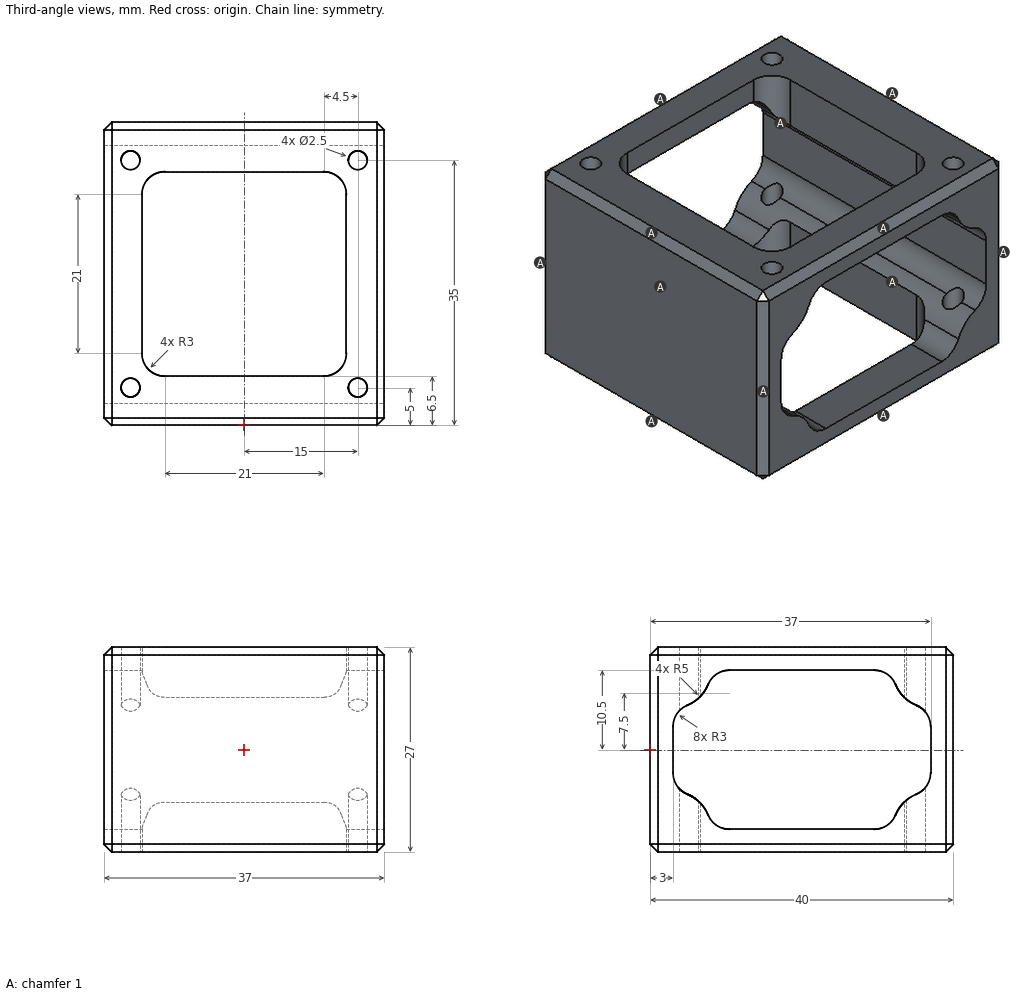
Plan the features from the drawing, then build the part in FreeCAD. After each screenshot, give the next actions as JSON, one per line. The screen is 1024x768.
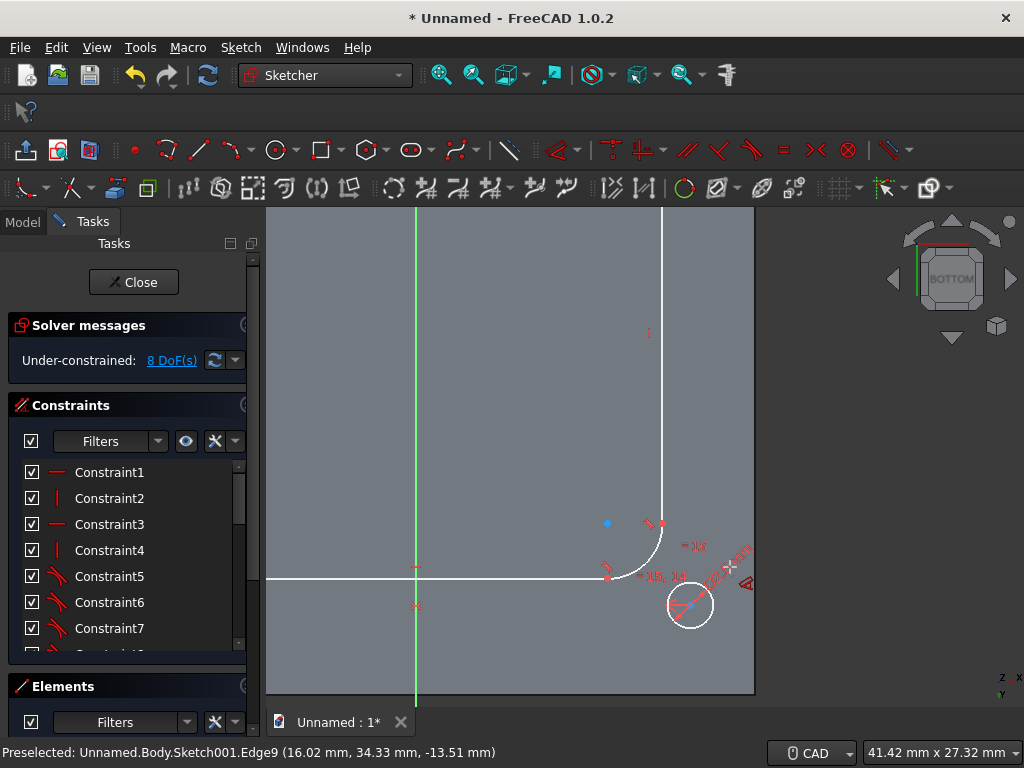
{"action": "scroll", "coordinate": [707, 589], "scroll_direction": "down", "scroll_amount": 4}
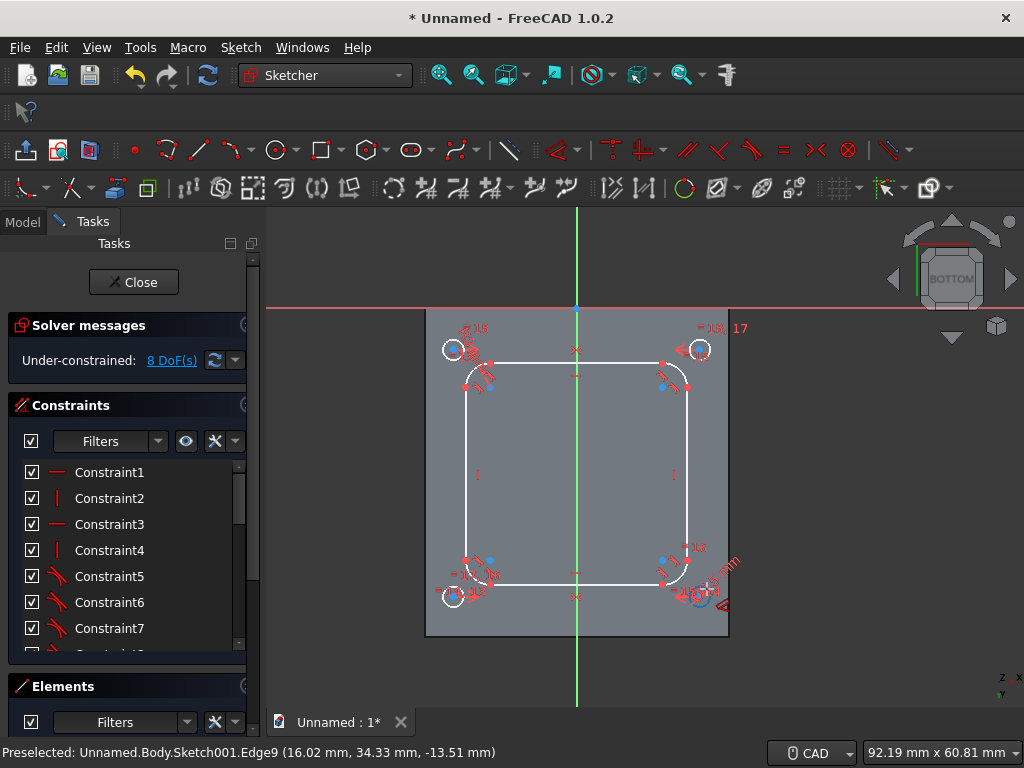
{"action": "left_click", "coordinate": [700, 350]}
{"action": "left_click", "coordinate": [734, 329]}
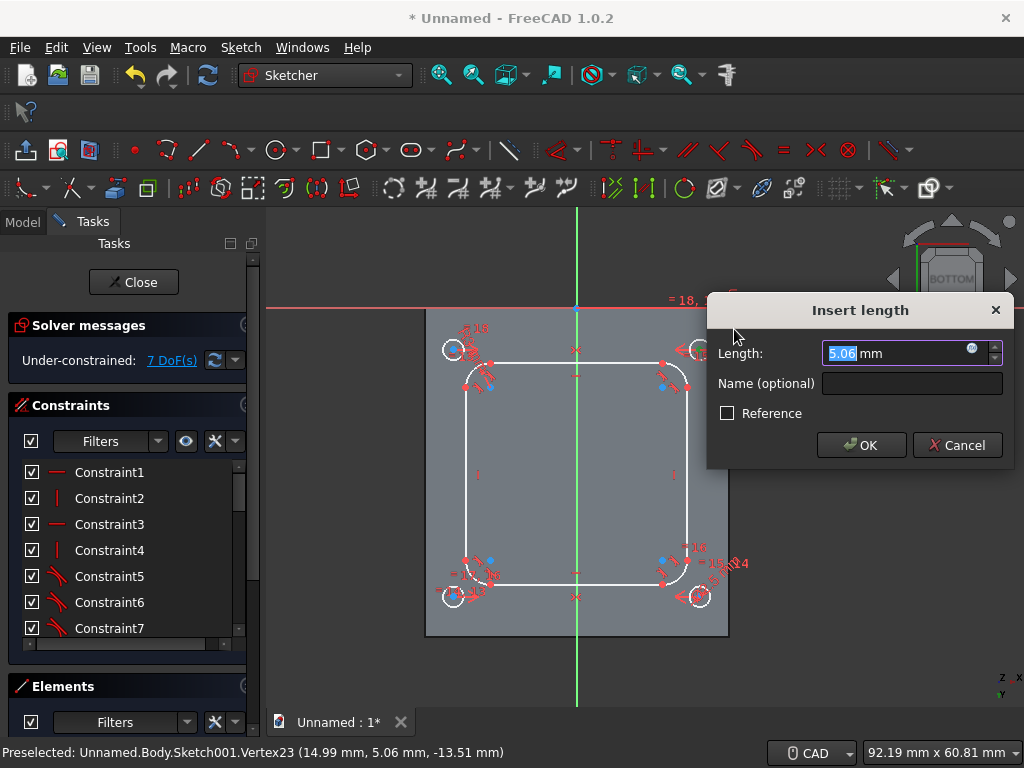
{"action": "type", "text": "5"}
{"action": "key", "text": "Return"}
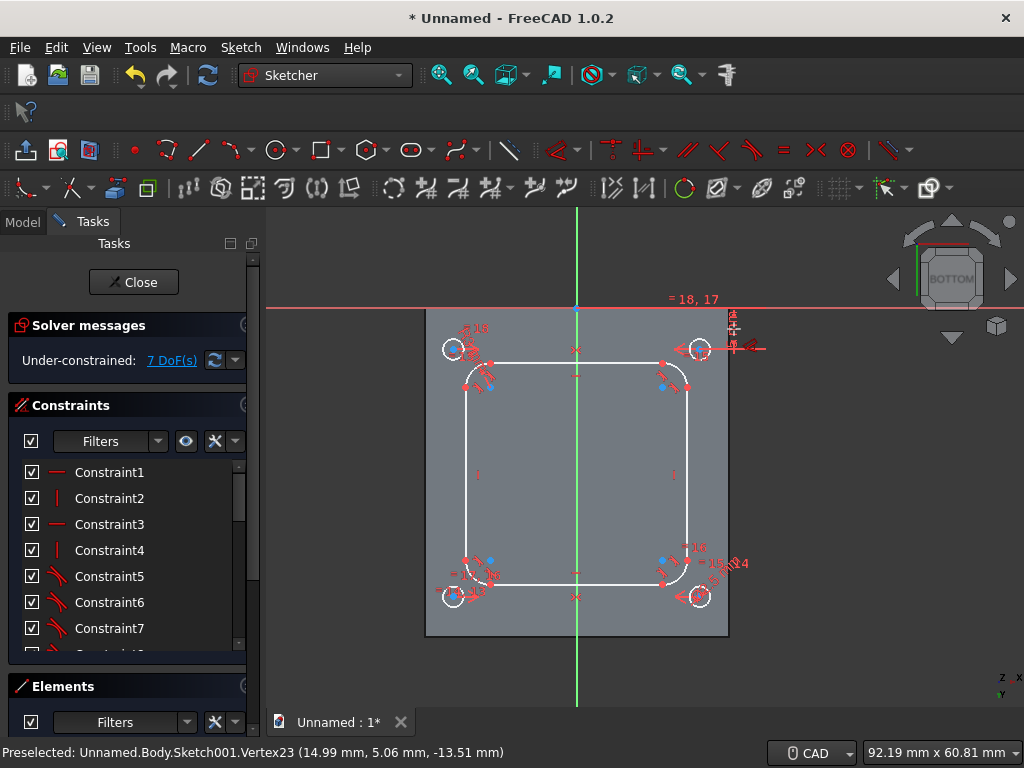
{"action": "left_click", "coordinate": [611, 363]}
{"action": "left_click", "coordinate": [537, 329]}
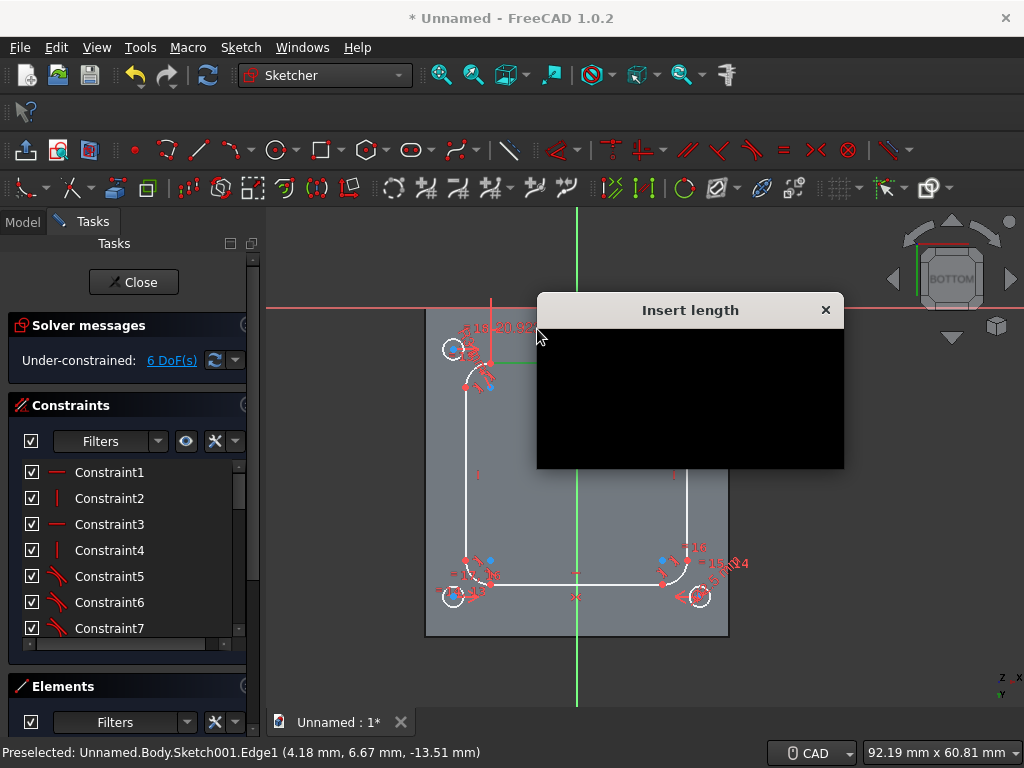
{"action": "type", "text": "21"}
{"action": "key", "text": "Return"}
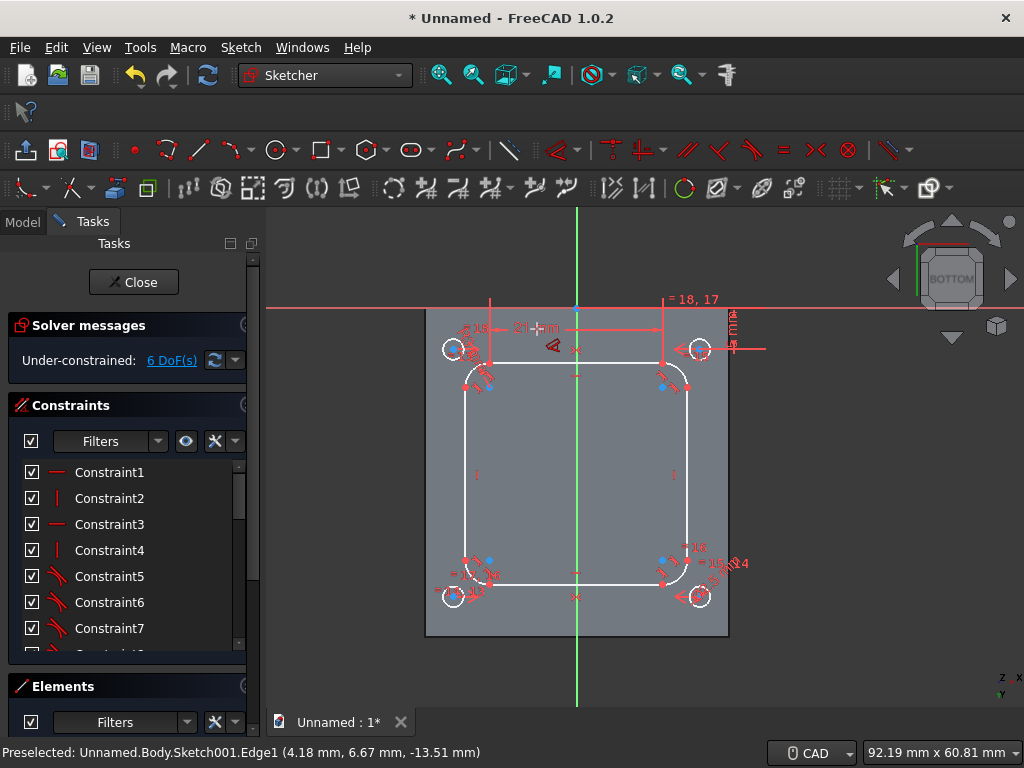
{"action": "left_click", "coordinate": [465, 440]}
{"action": "left_click", "coordinate": [431, 474]}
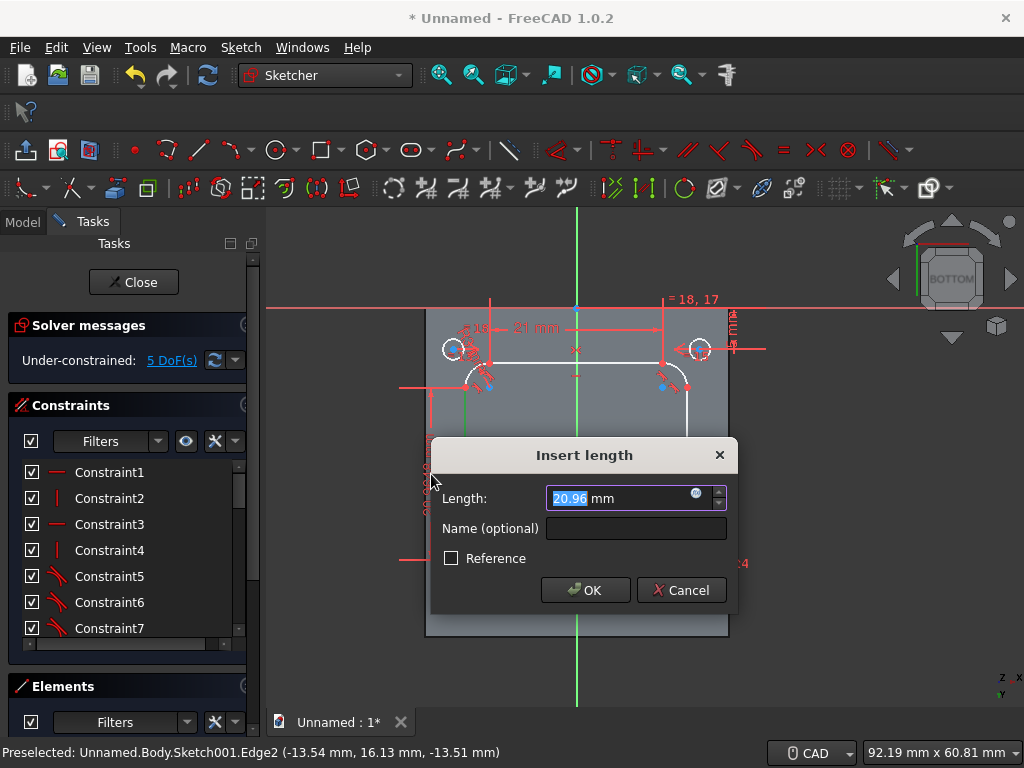
{"action": "type", "text": "21"}
{"action": "key", "text": "Return"}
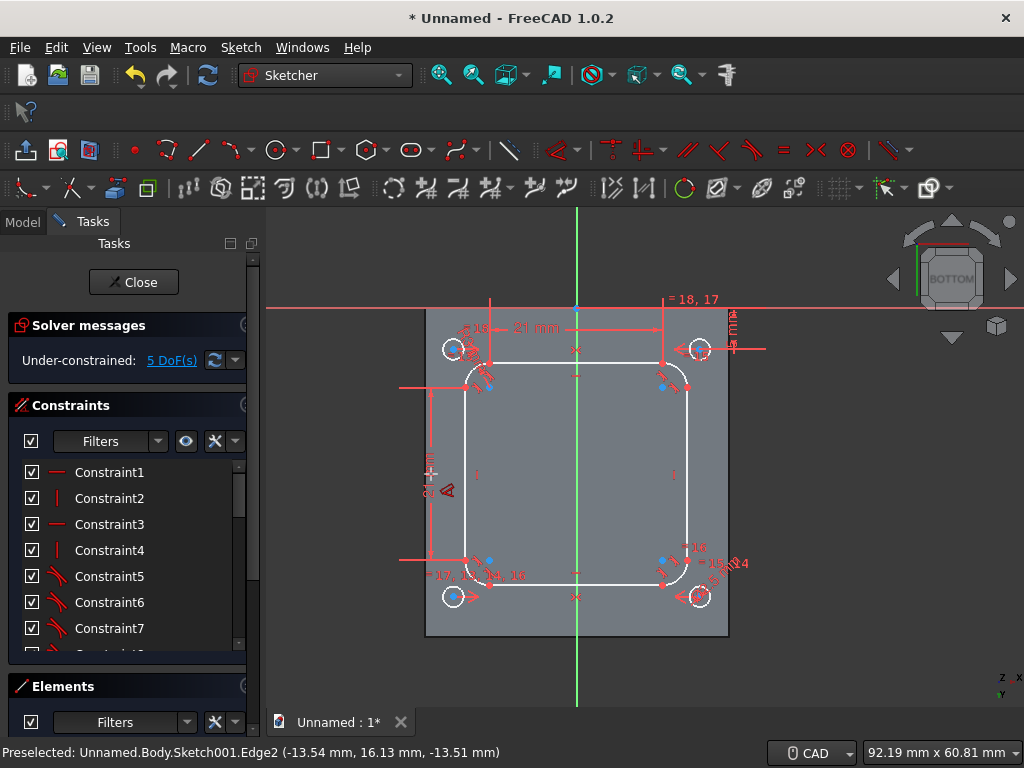
{"action": "left_click", "coordinate": [700, 597]}
{"action": "left_click", "coordinate": [638, 274]}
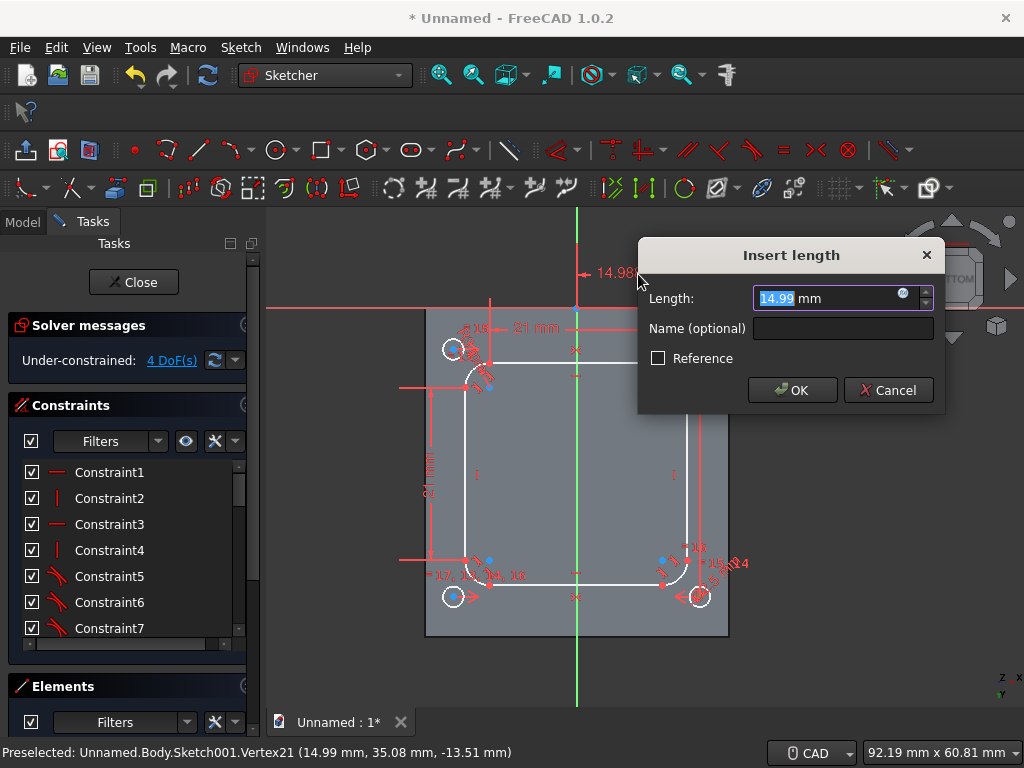
{"action": "type", "text": "15"}
{"action": "key", "text": "Return"}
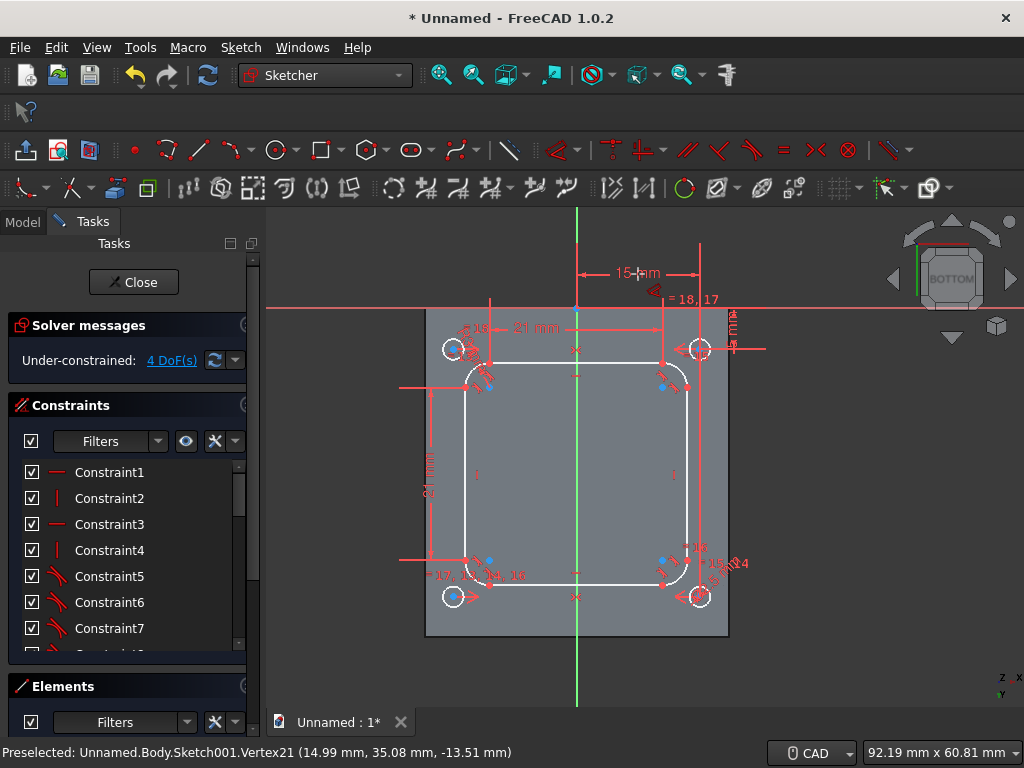
{"action": "left_click", "coordinate": [700, 597]}
{"action": "left_click", "coordinate": [734, 453]}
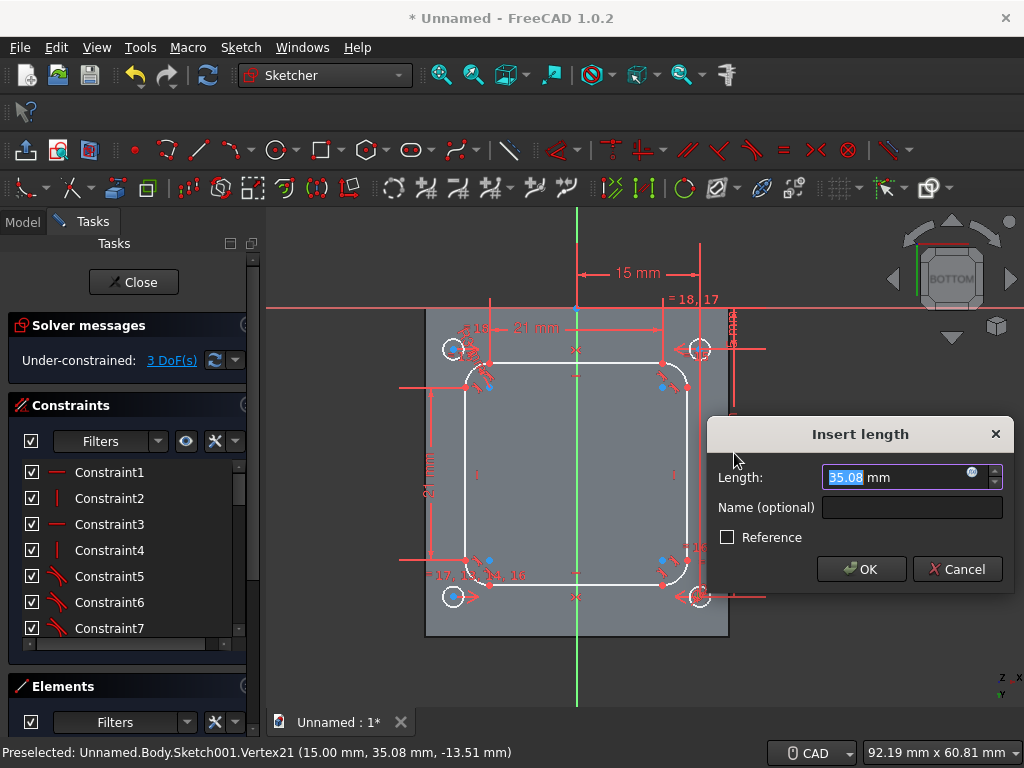
{"action": "type", "text": "35"}
{"action": "key", "text": "Return"}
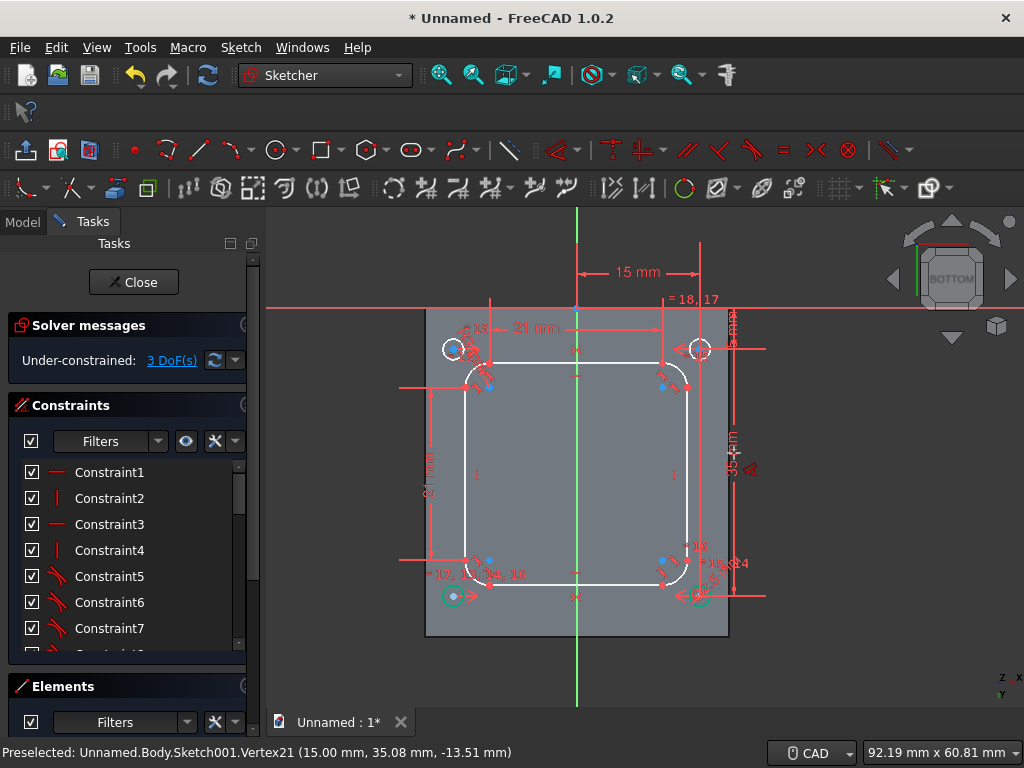
{"action": "left_click", "coordinate": [700, 349]}
{"action": "left_click", "coordinate": [638, 383]}